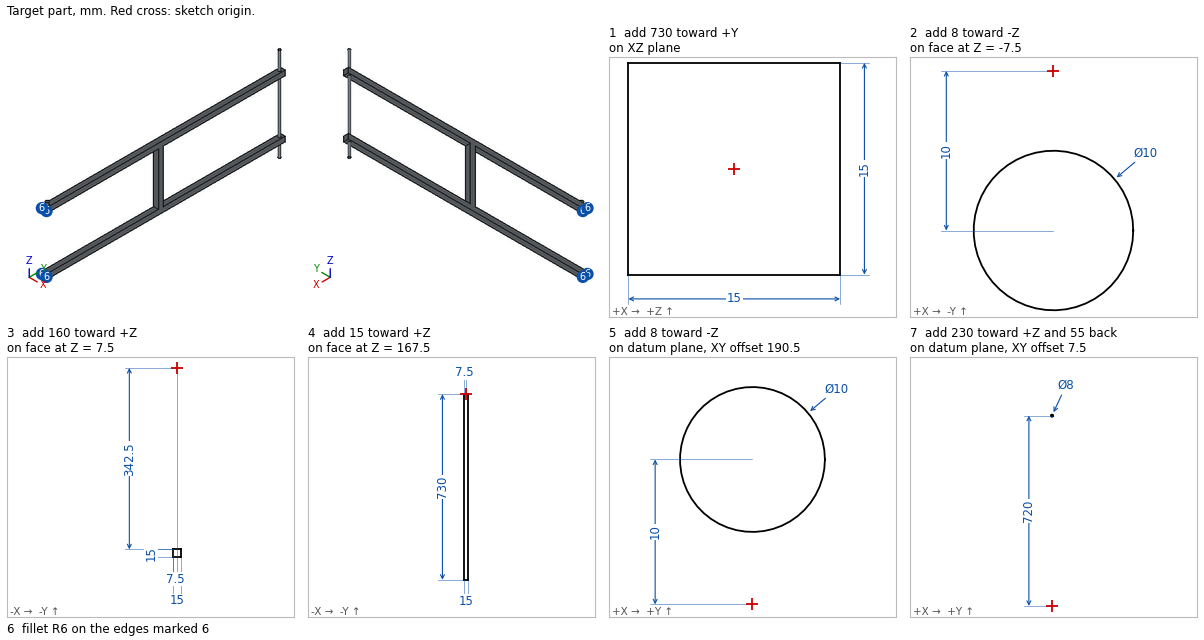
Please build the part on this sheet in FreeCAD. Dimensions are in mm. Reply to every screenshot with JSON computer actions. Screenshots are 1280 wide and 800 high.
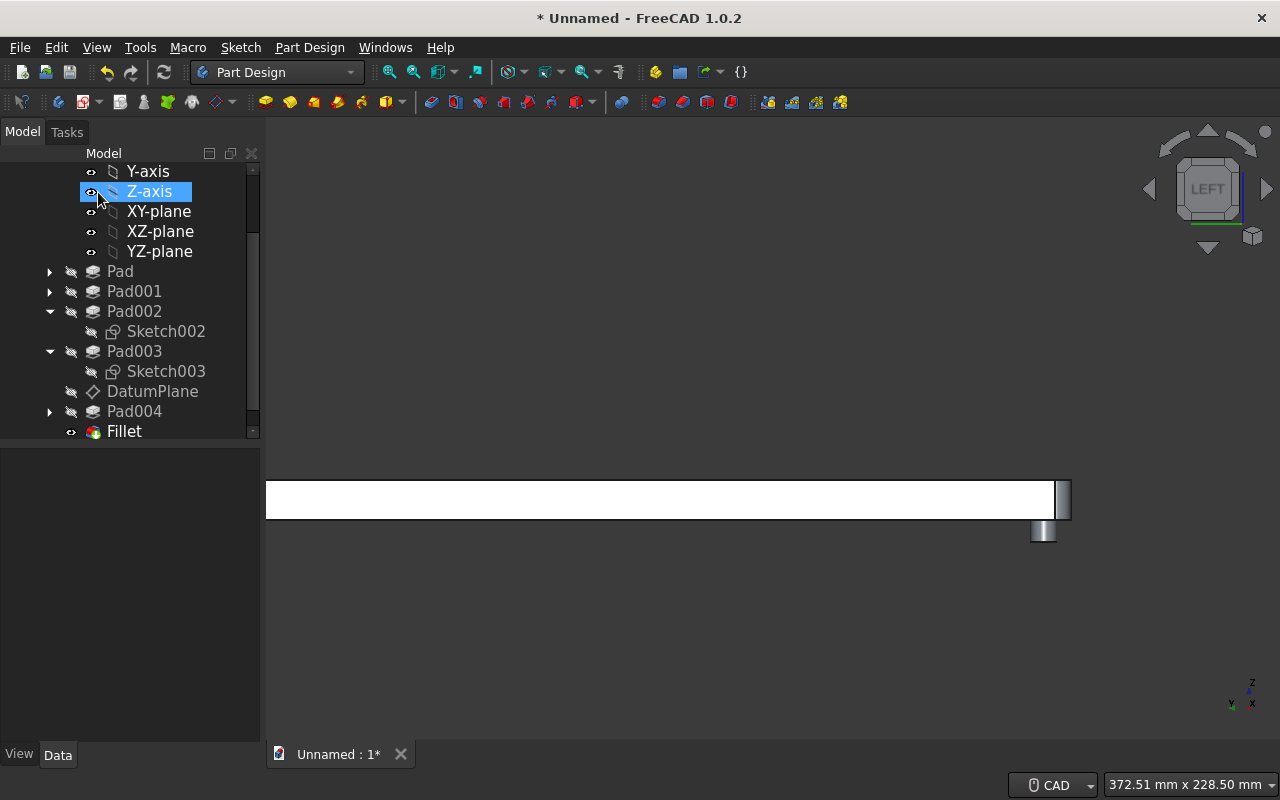
{"action": "left_click", "coordinate": [390, 72]}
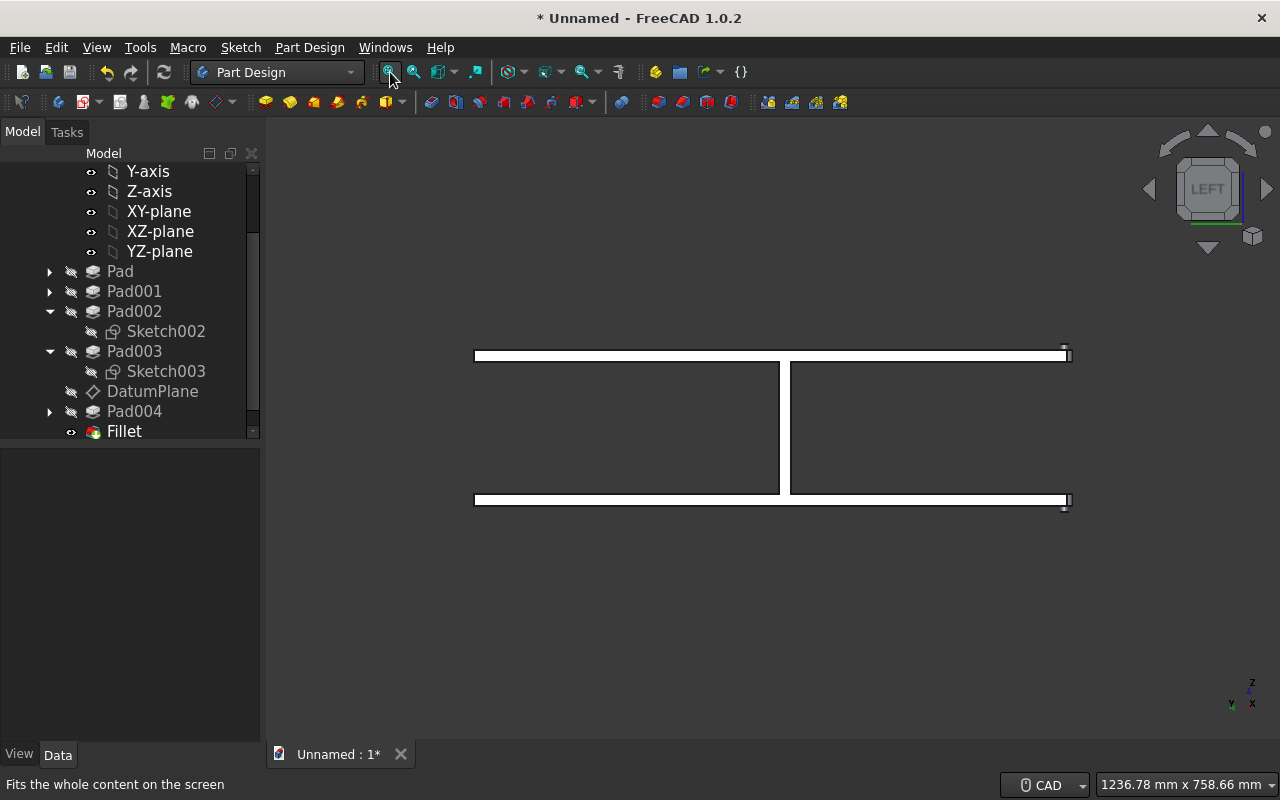
{"action": "scroll", "coordinate": [160, 307], "scroll_direction": "down", "scroll_amount": 3}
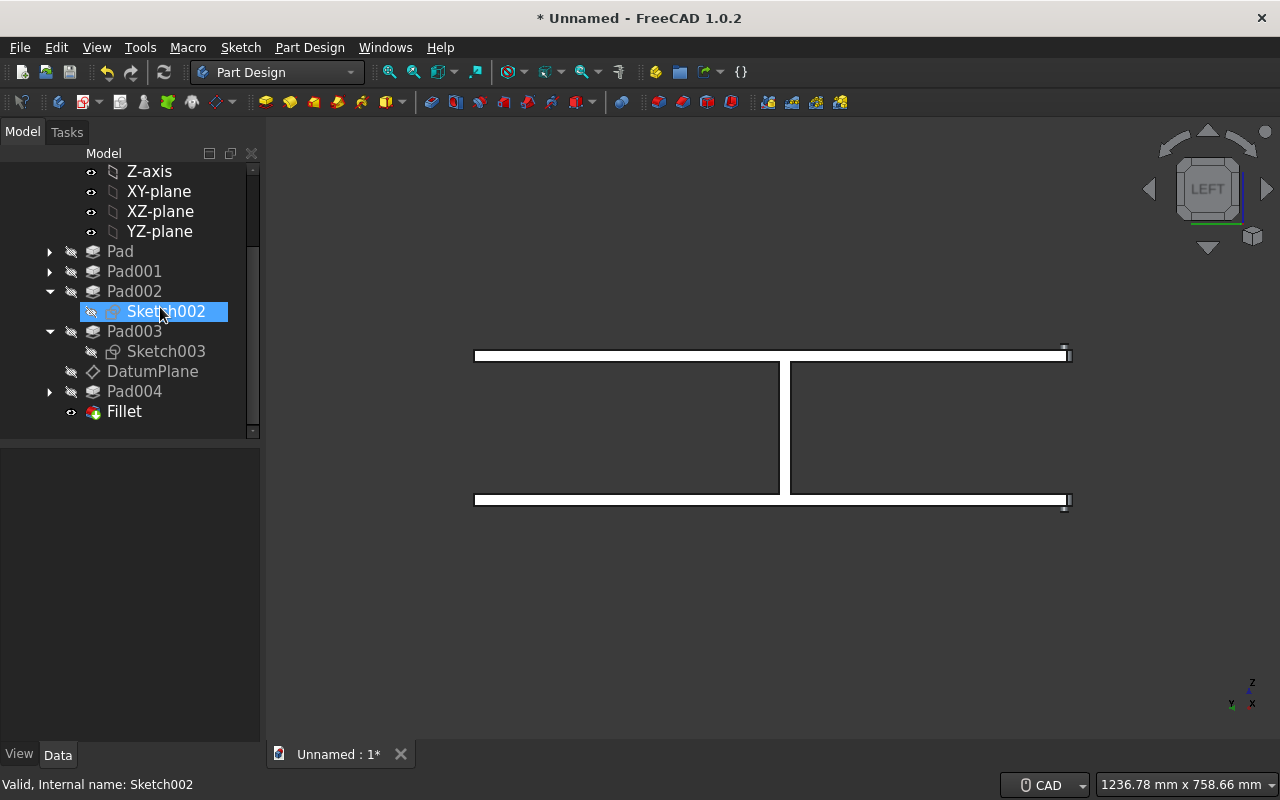
{"action": "scroll", "coordinate": [160, 287], "scroll_direction": "up", "scroll_amount": 15}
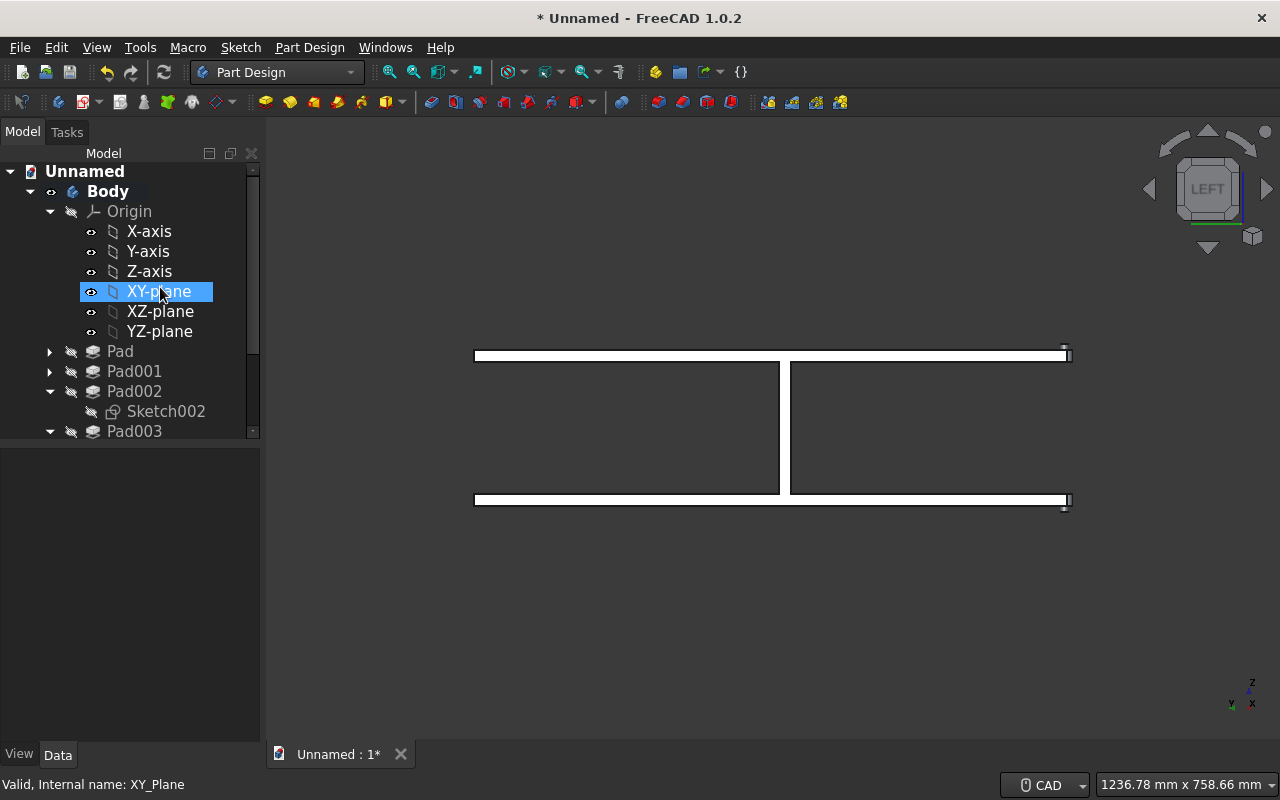
{"action": "left_click", "coordinate": [136, 292]}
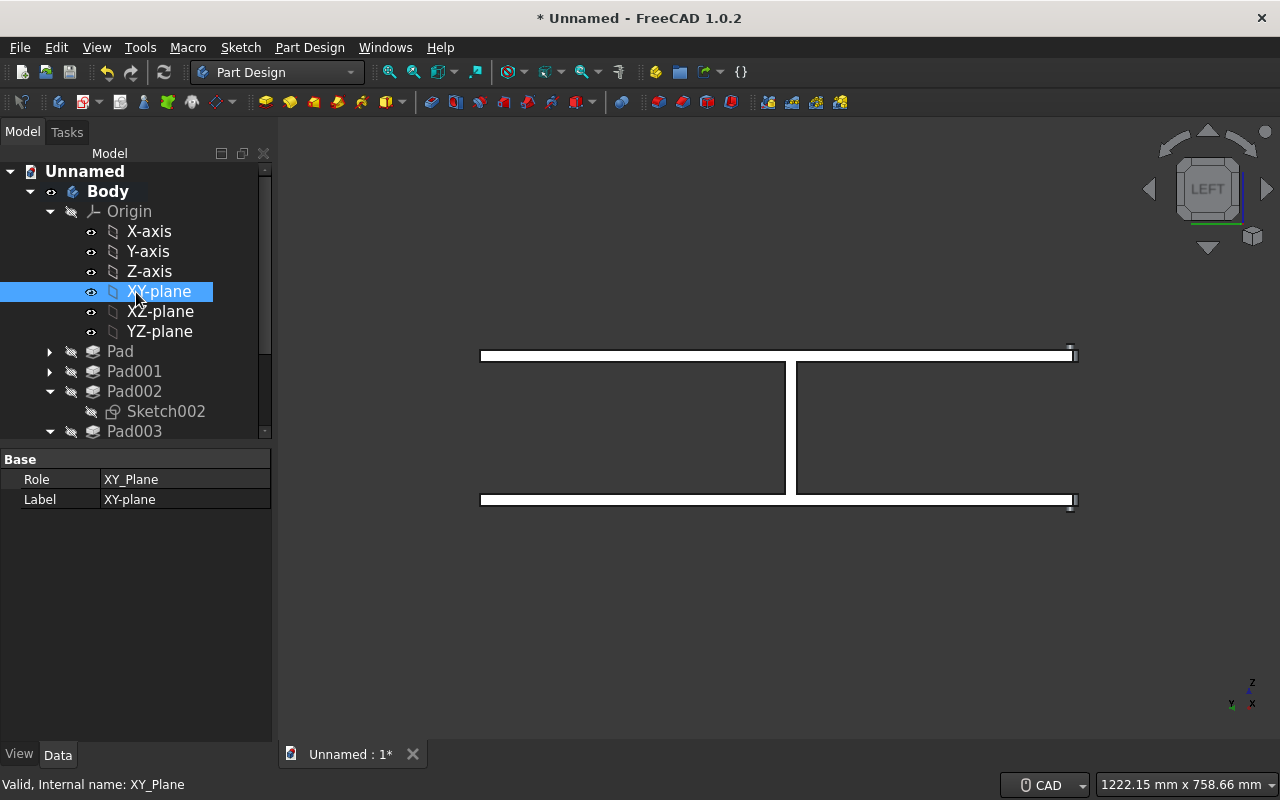
{"action": "left_click", "coordinate": [216, 102]}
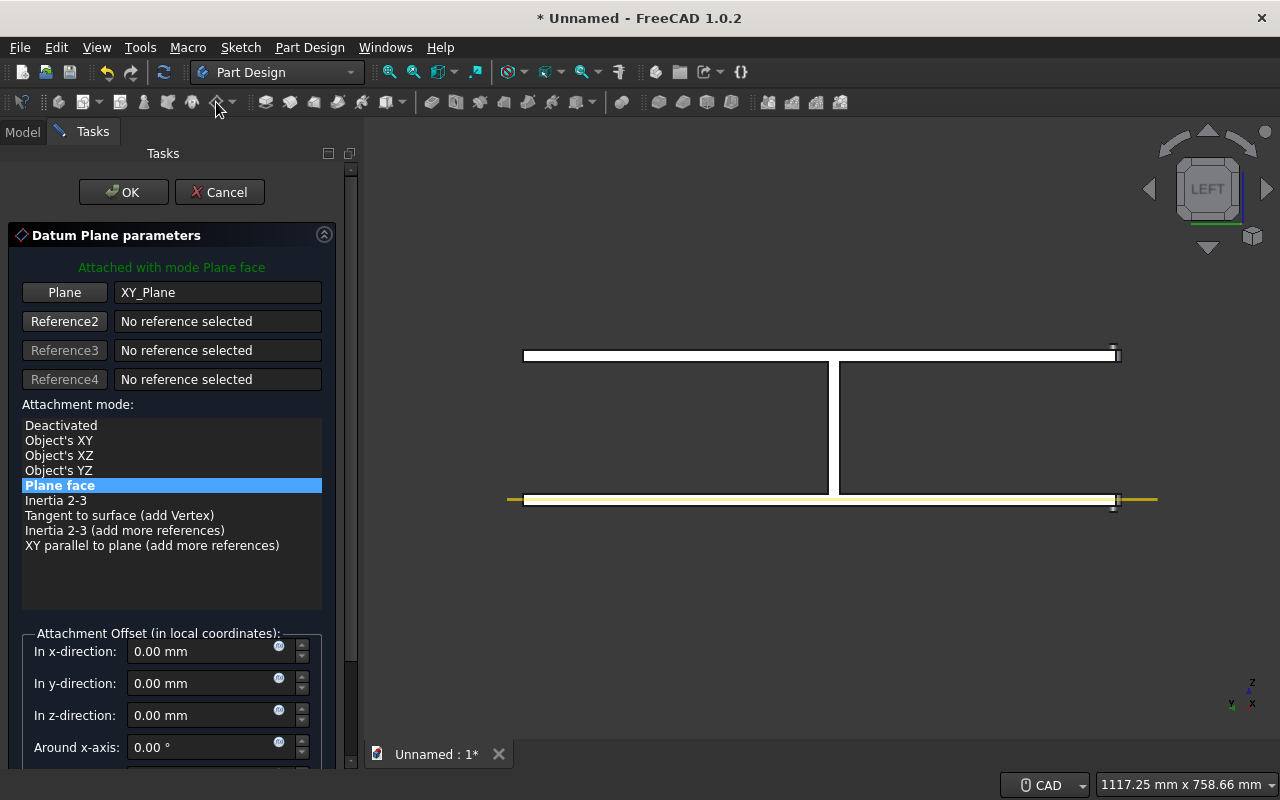
{"action": "triple_click", "coordinate": [210, 715]}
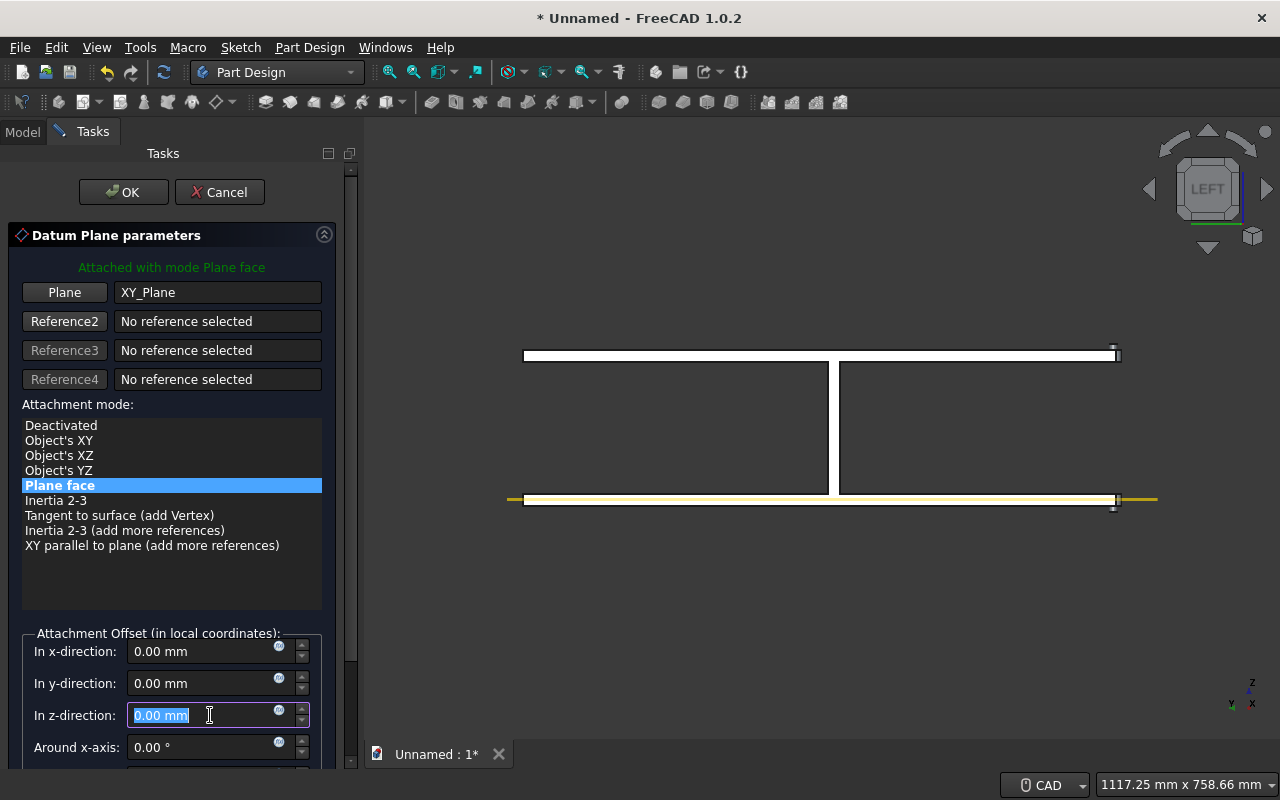
{"action": "type", "text": "7.5"}
{"action": "key", "text": "Tab"}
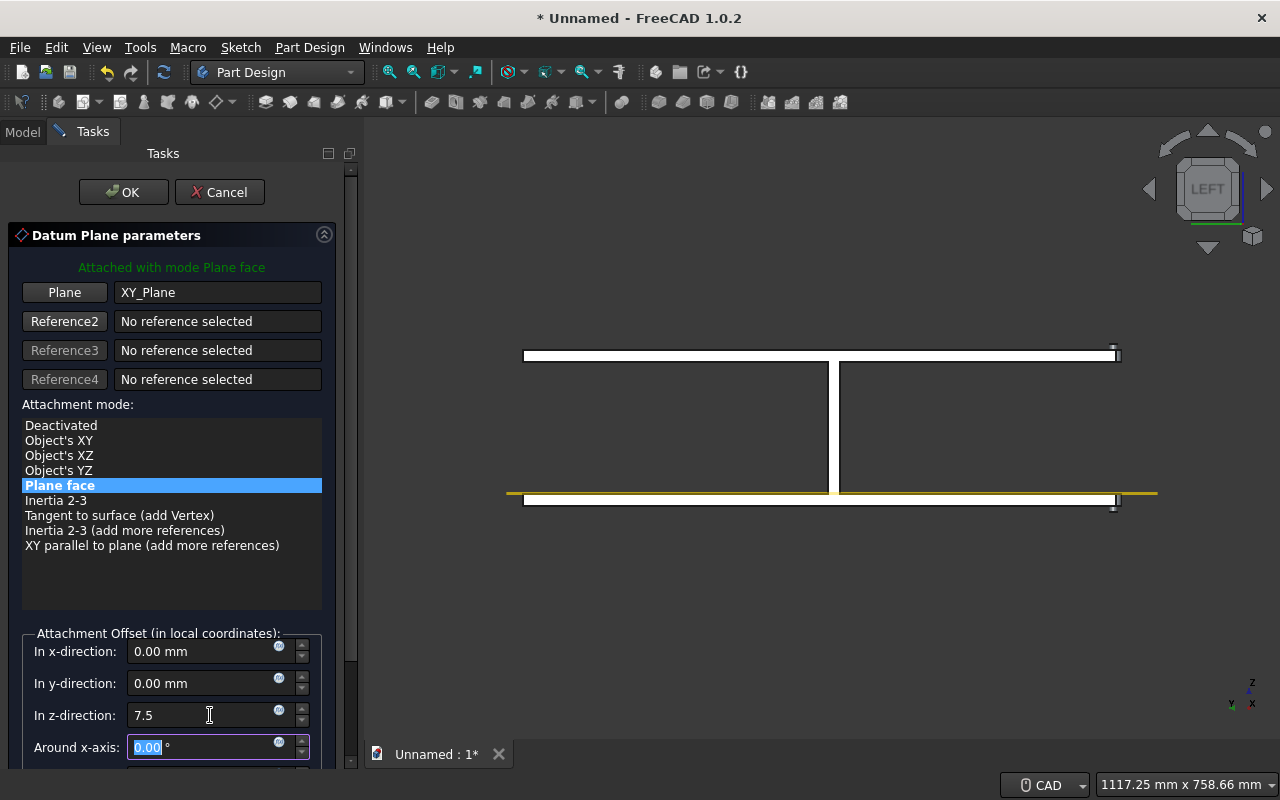
{"action": "left_click", "coordinate": [124, 192]}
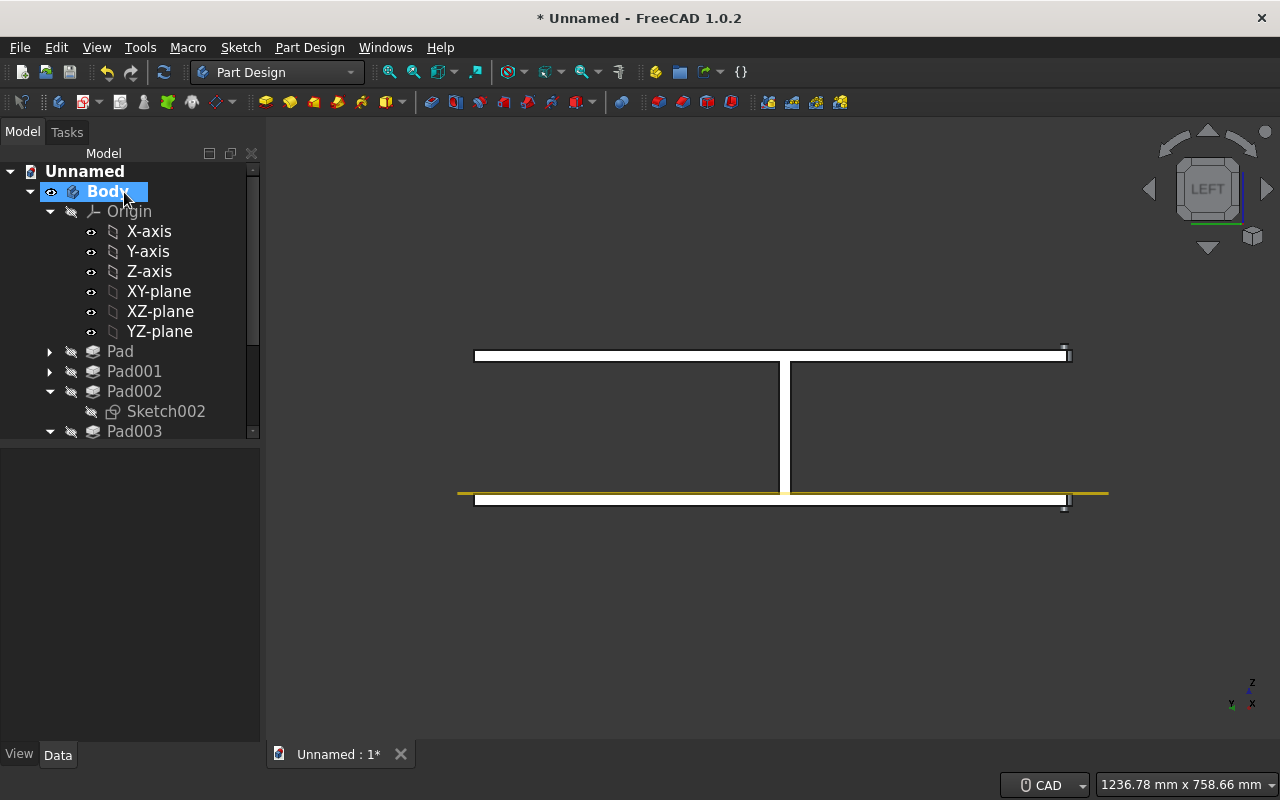
{"action": "scroll", "coordinate": [100, 307], "scroll_direction": "down", "scroll_amount": 3}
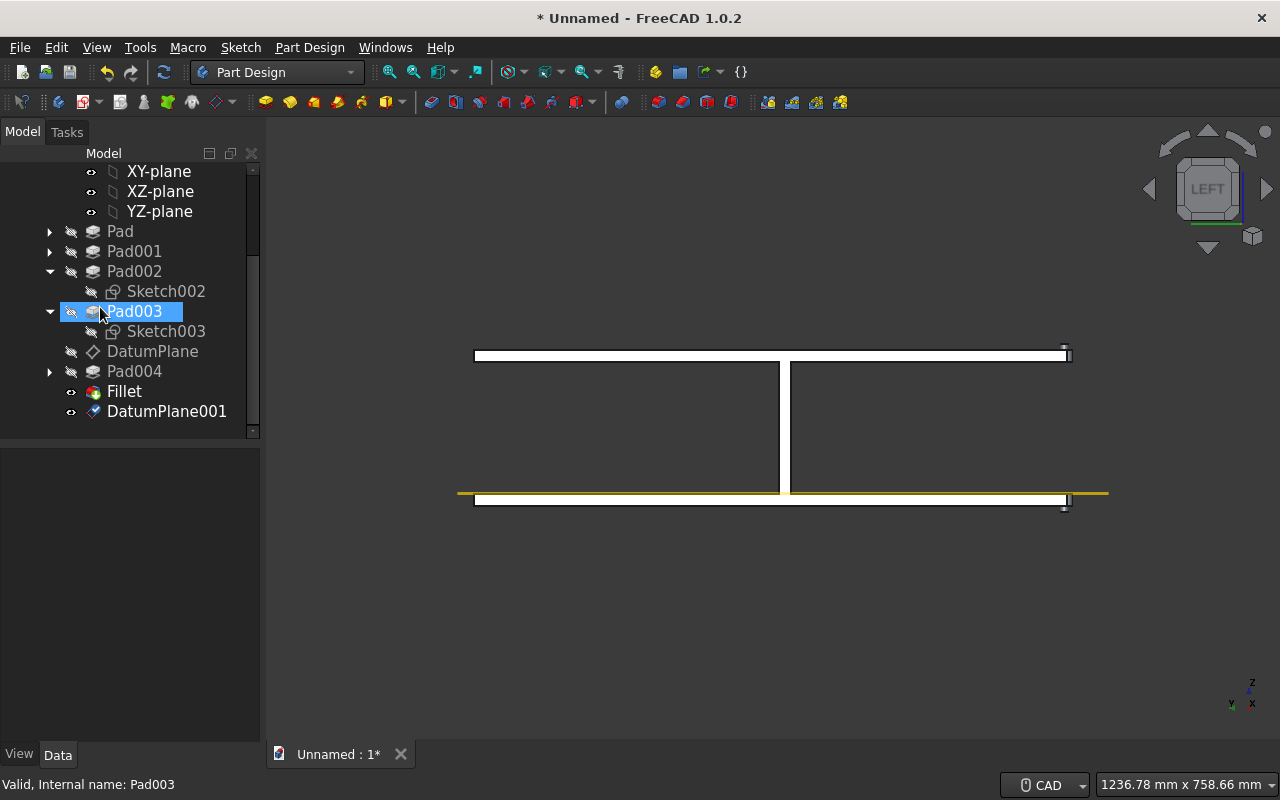
{"action": "left_click", "coordinate": [116, 412]}